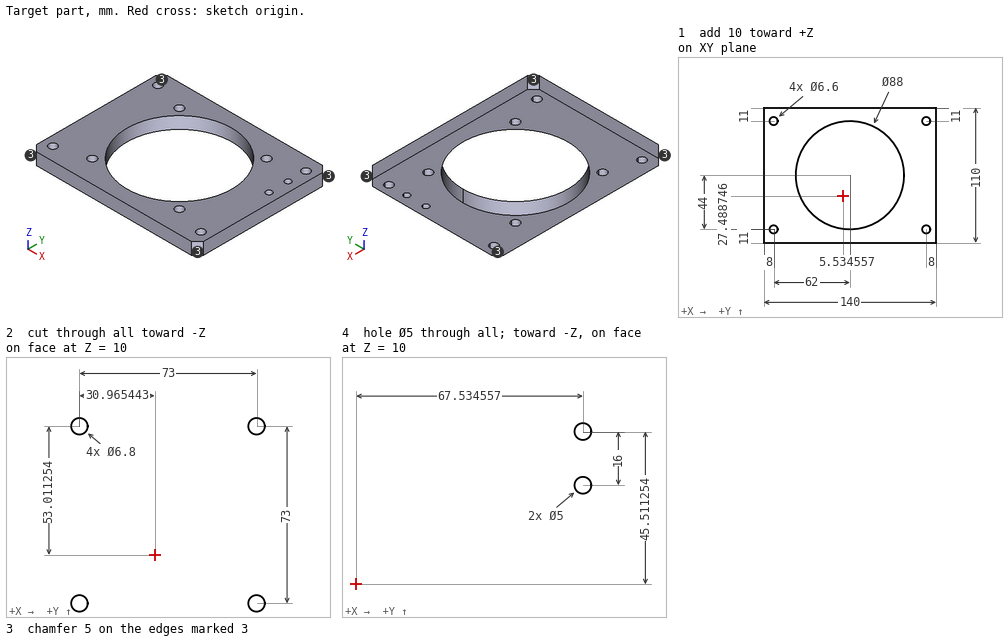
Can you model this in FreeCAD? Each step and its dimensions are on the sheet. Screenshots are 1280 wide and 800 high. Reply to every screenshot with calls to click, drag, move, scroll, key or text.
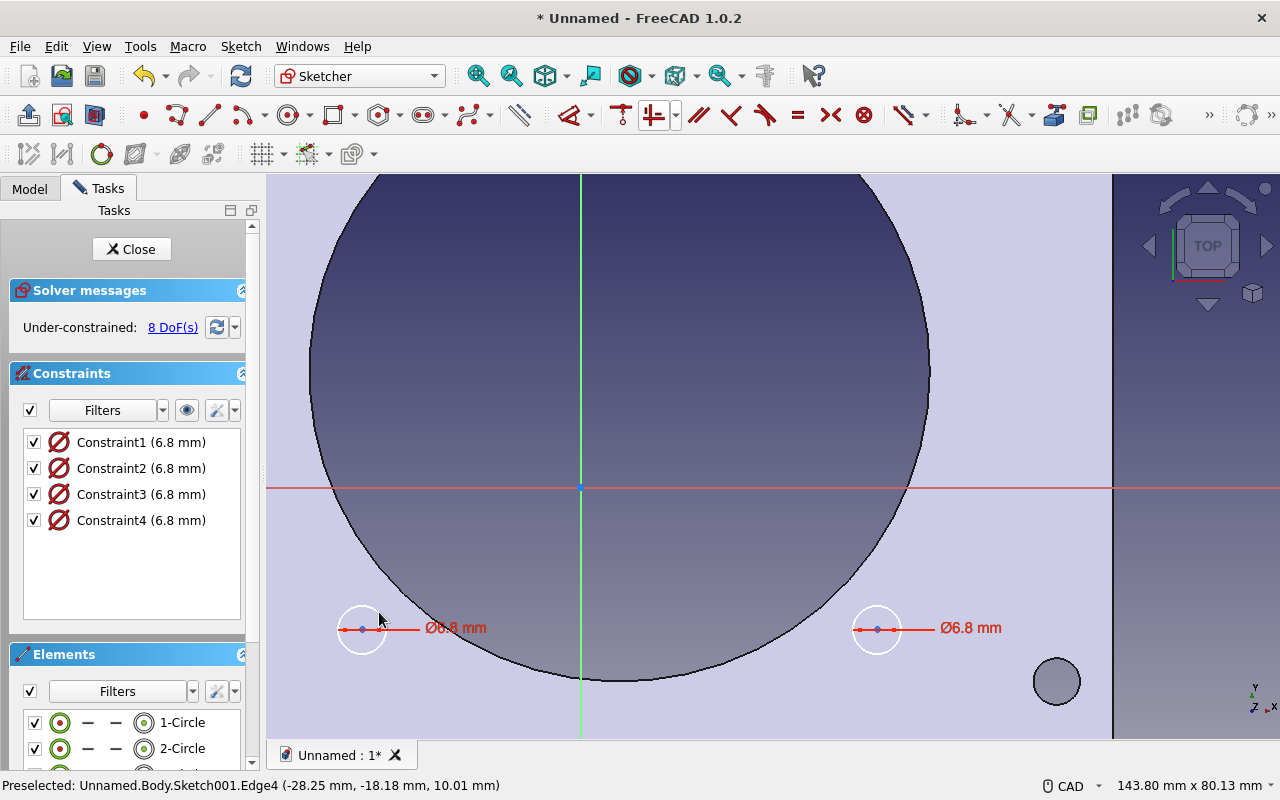
scroll(877, 630, down, 2)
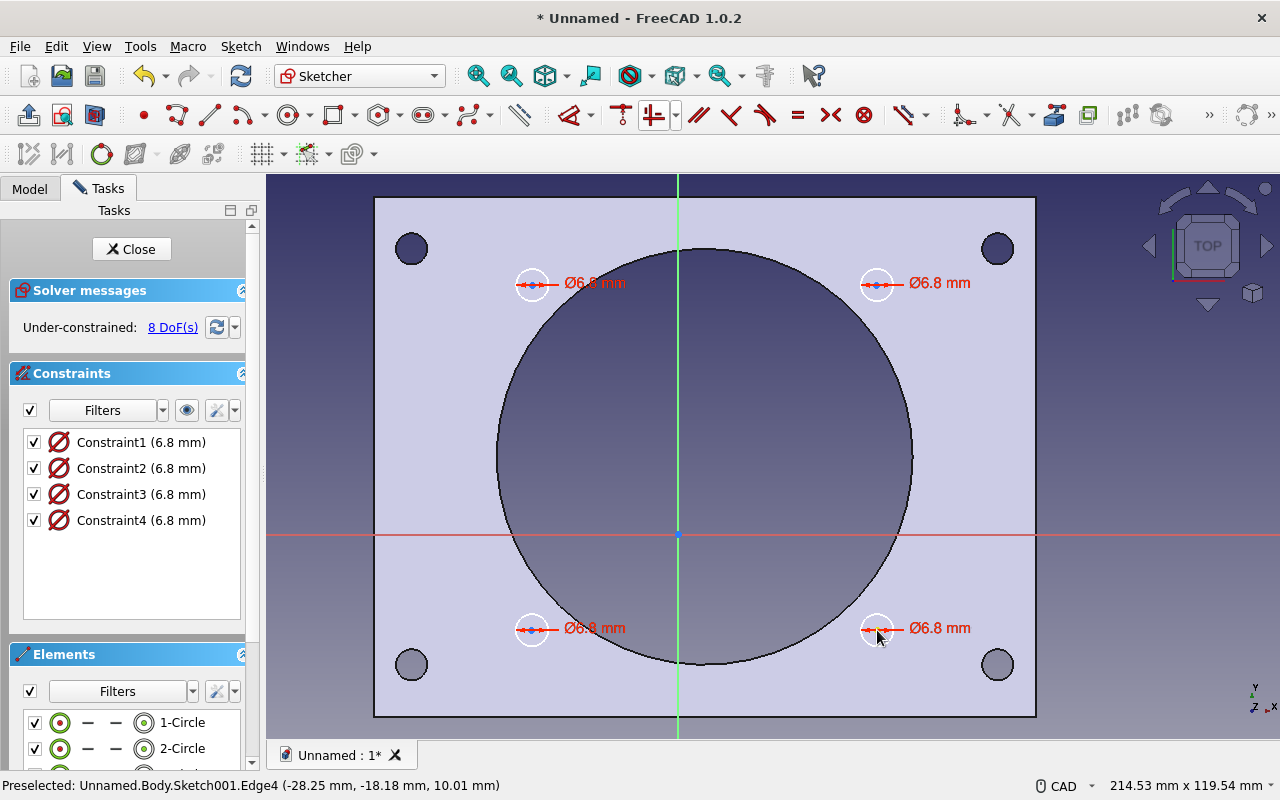
click(532, 285)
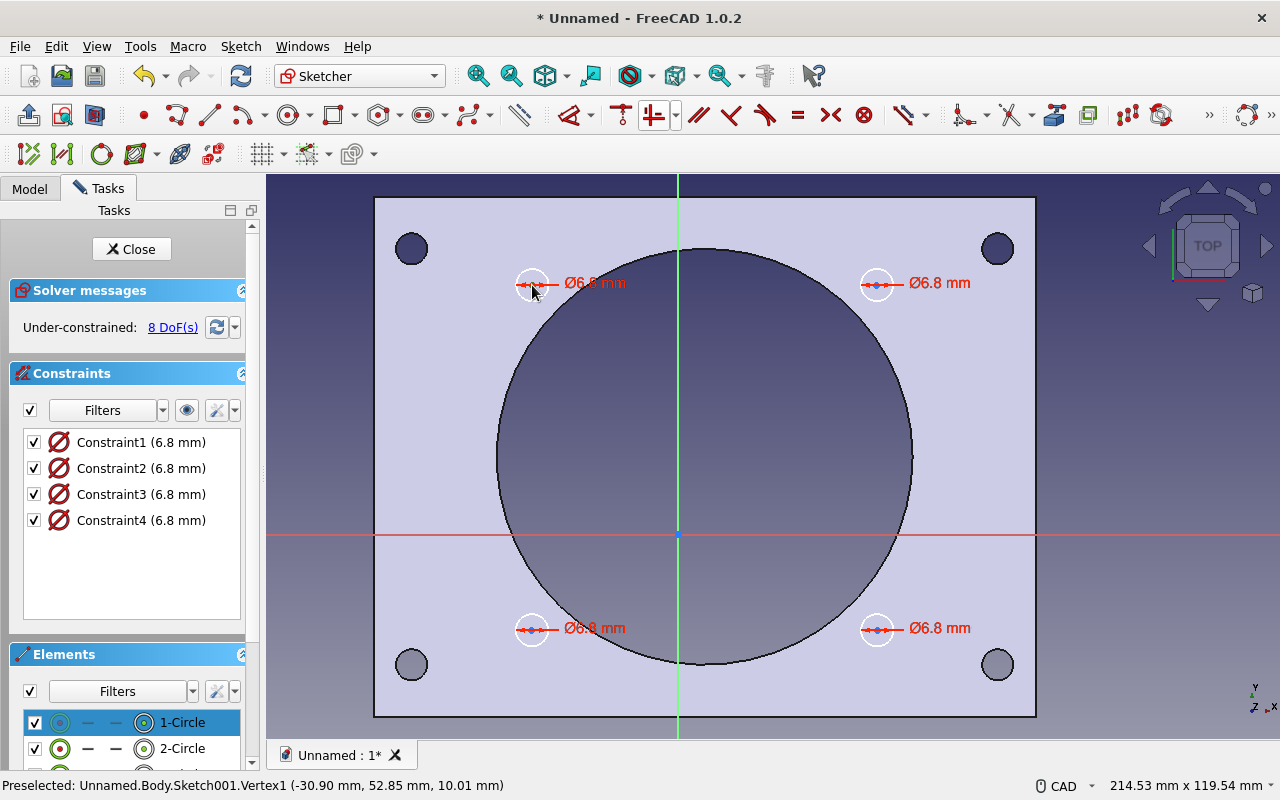
click(877, 285)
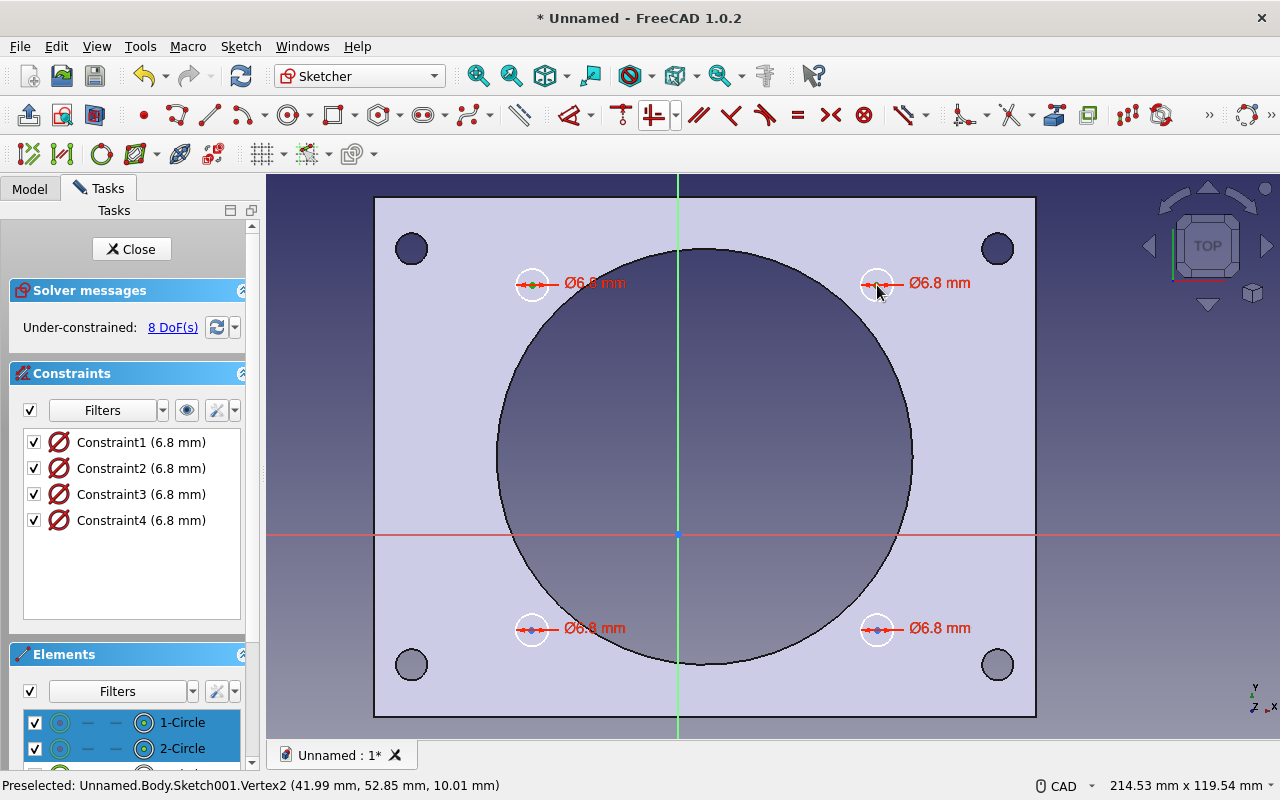
click(676, 116)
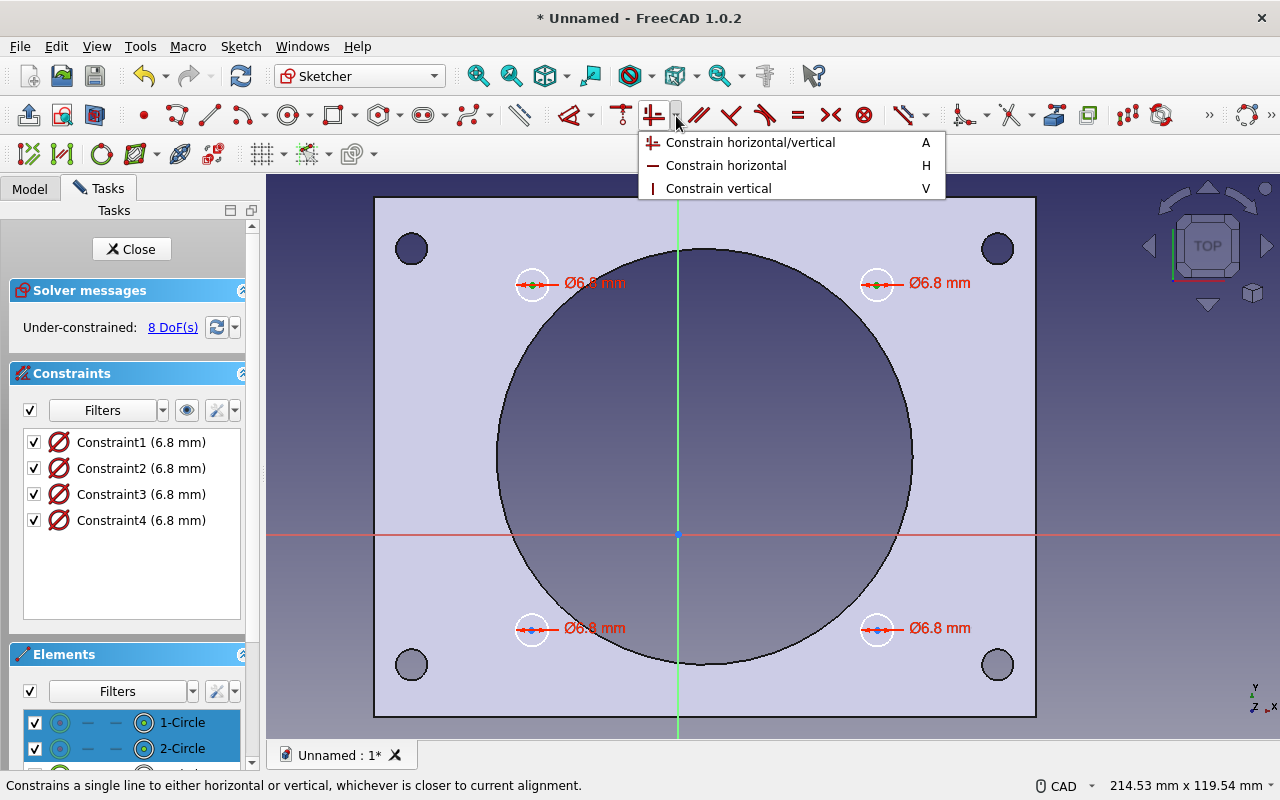
click(792, 166)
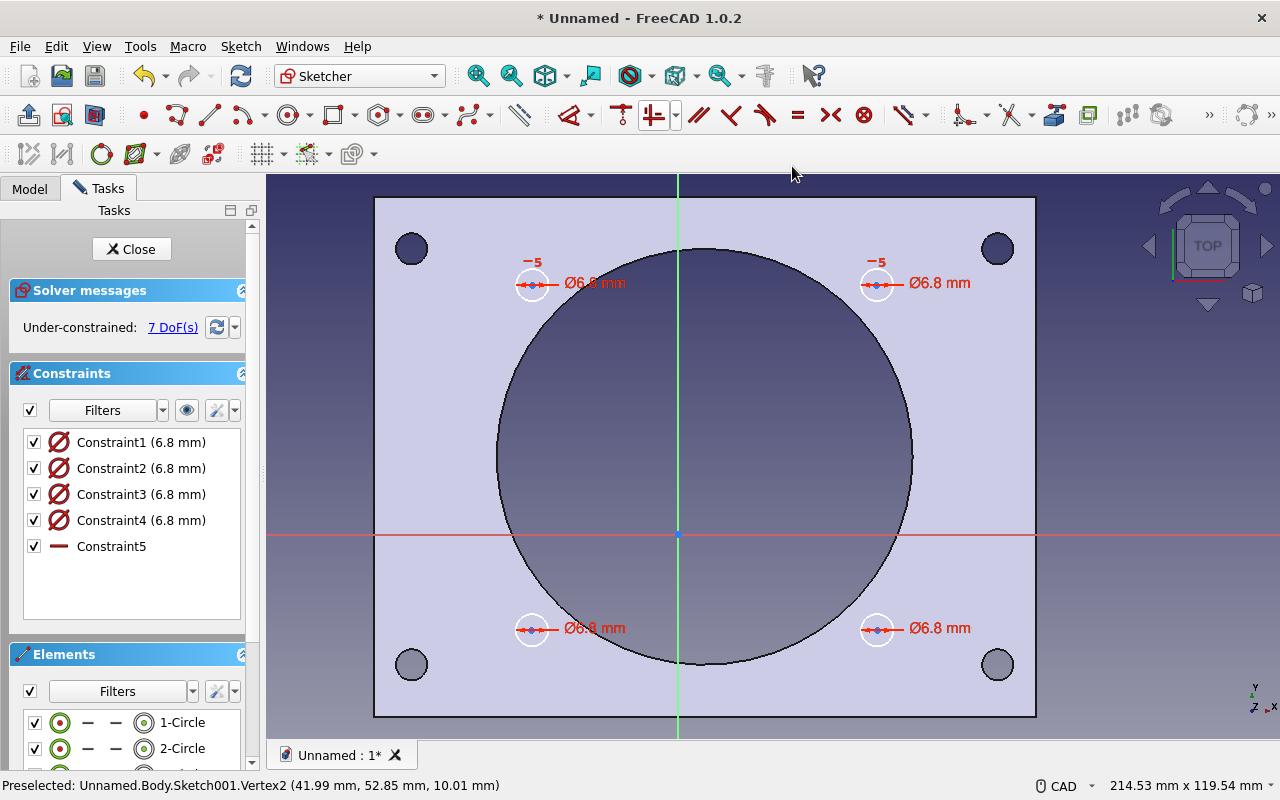
click(877, 285)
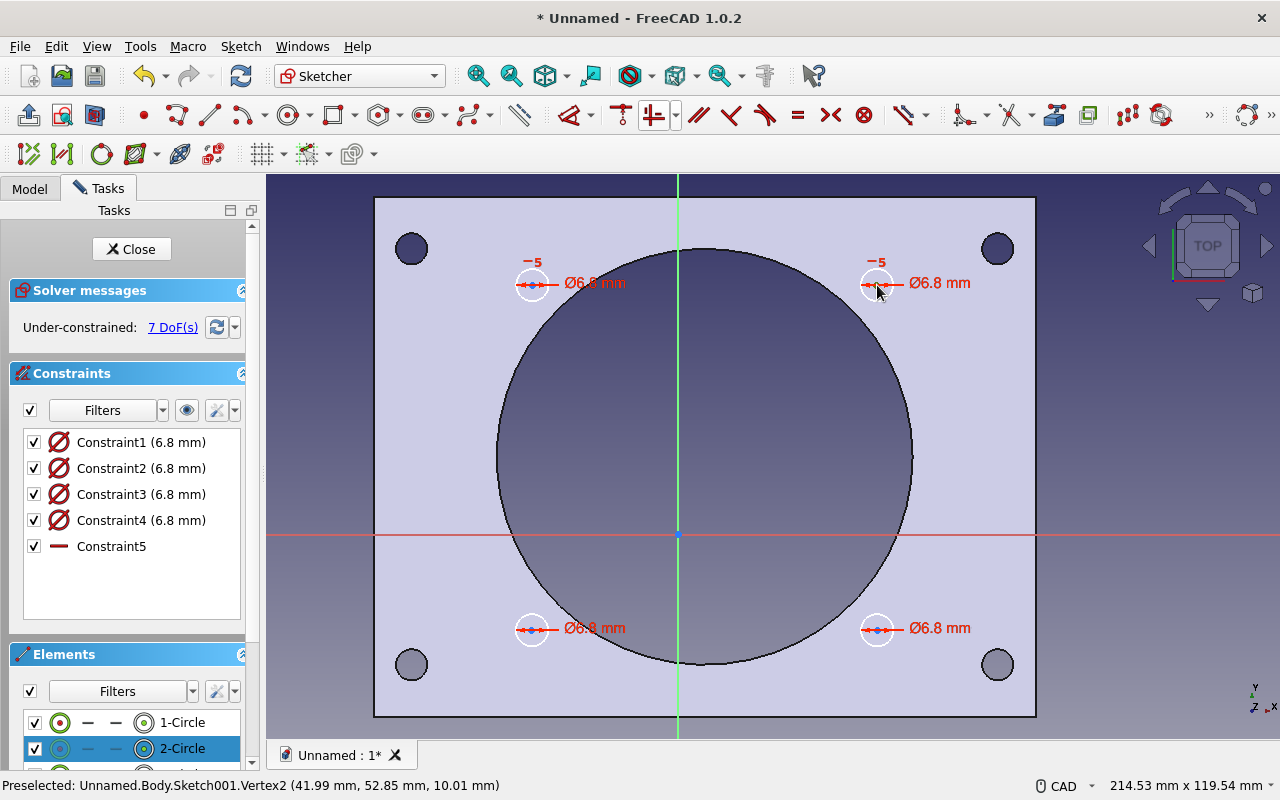
click(877, 630)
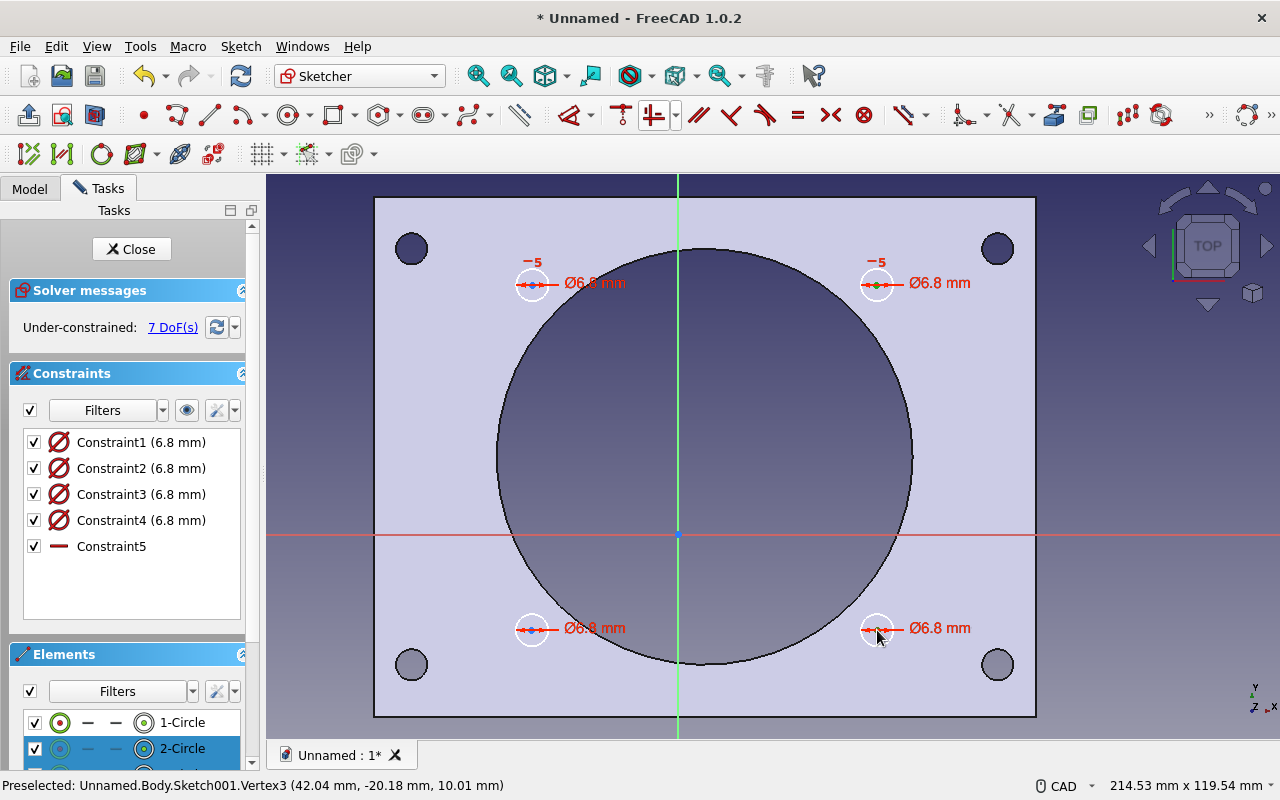
click(676, 116)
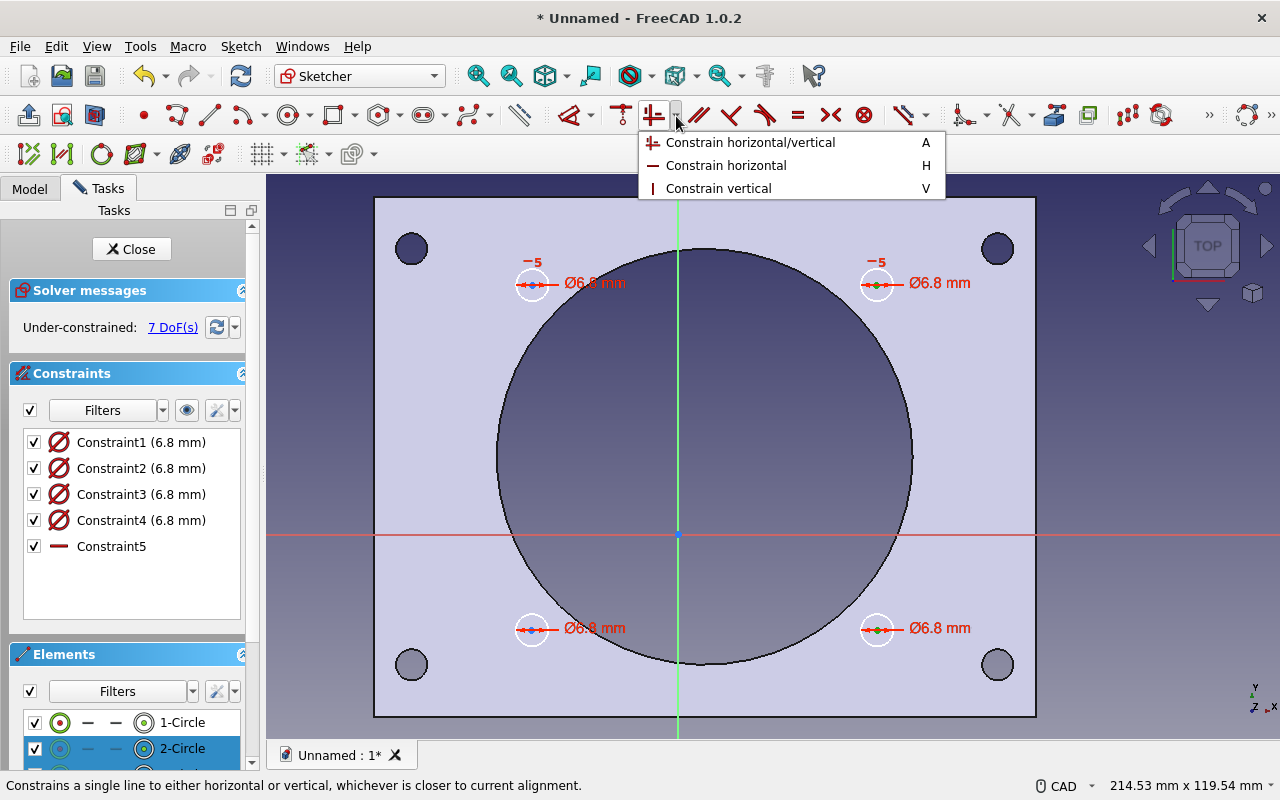
click(792, 188)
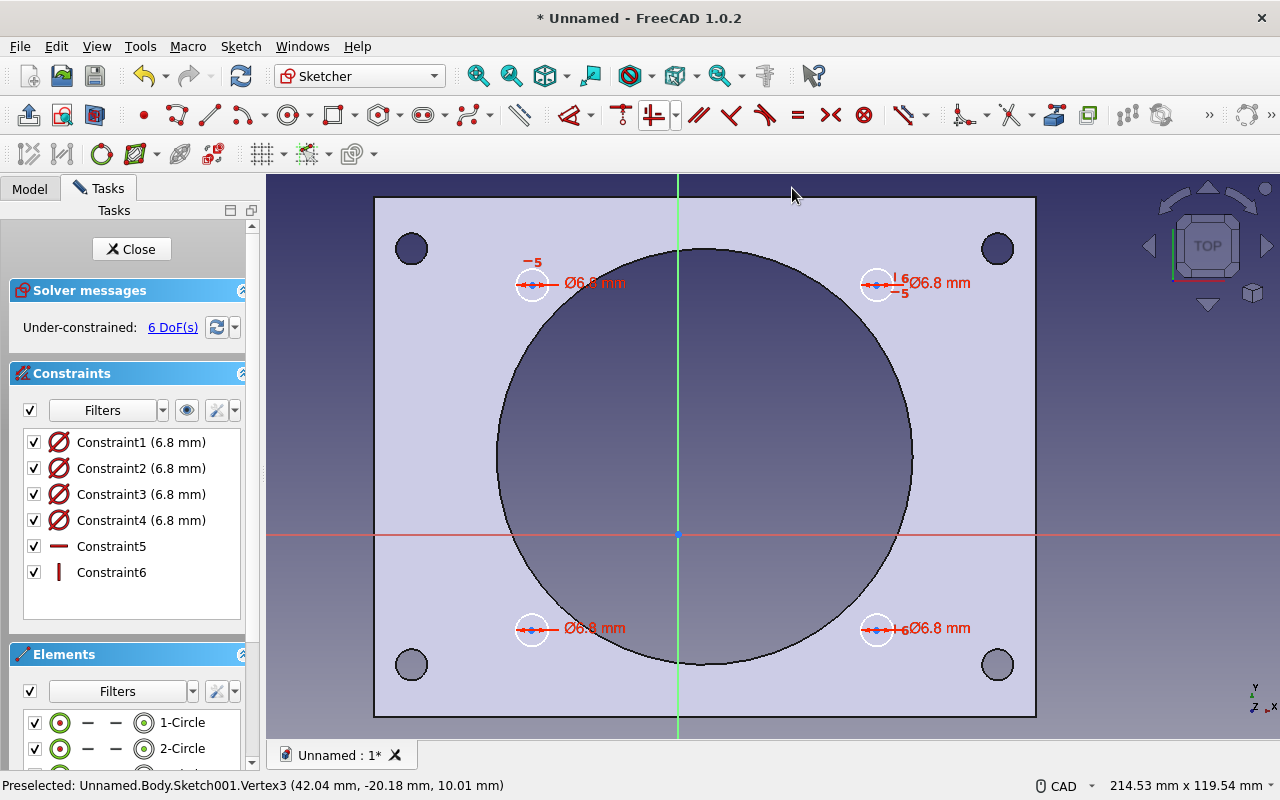
click(532, 285)